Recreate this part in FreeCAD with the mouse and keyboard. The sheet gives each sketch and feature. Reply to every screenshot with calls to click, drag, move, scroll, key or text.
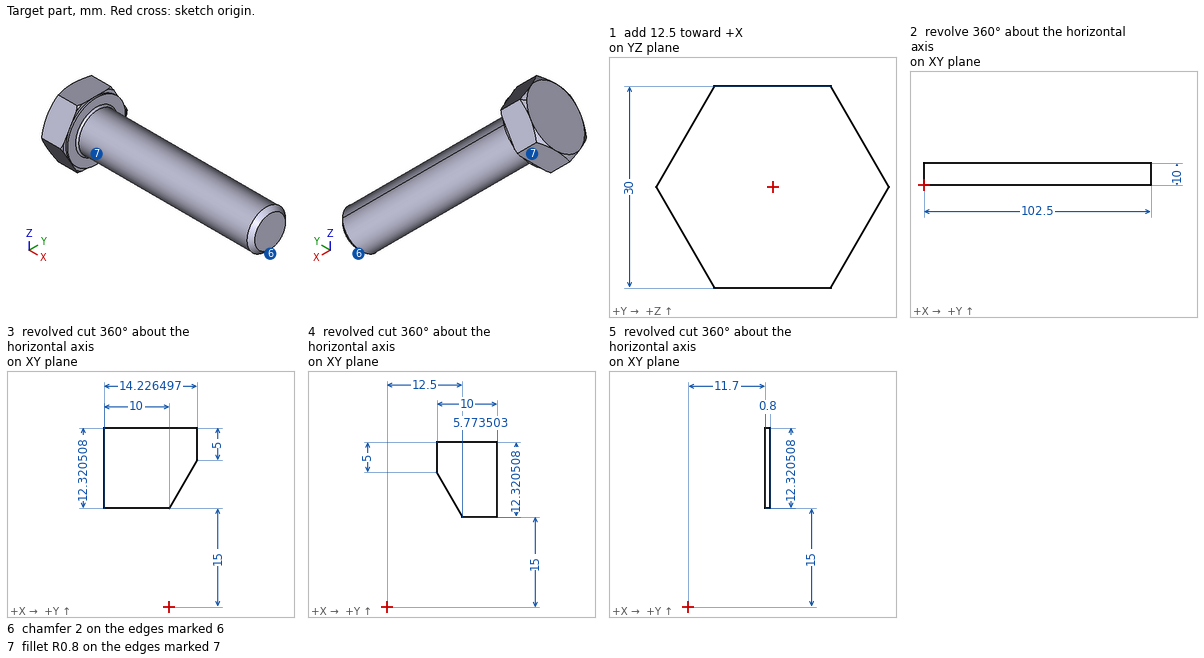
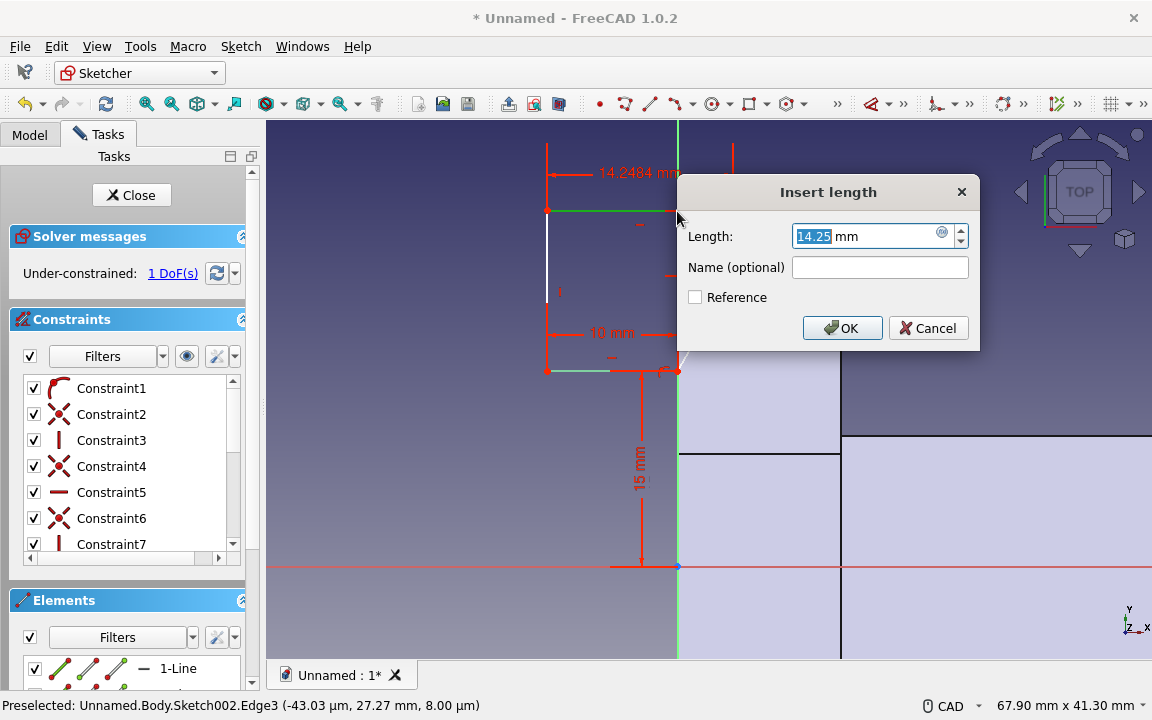
text(14.226497)
key(Return)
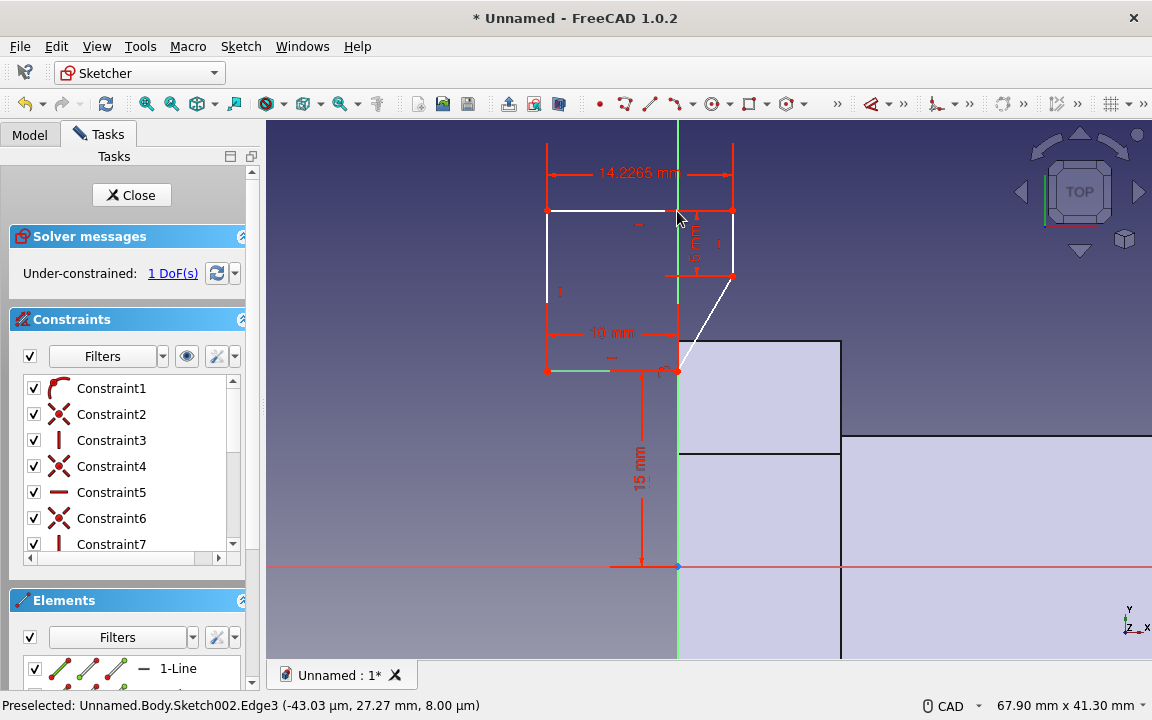
click(547, 259)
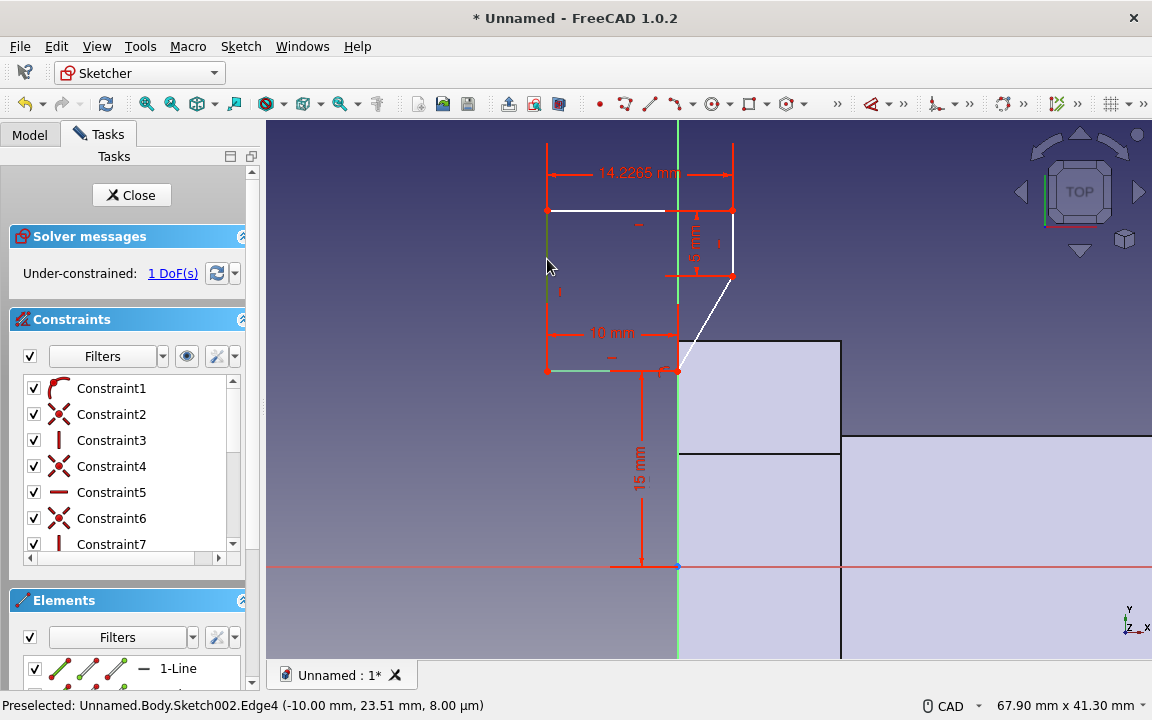
key(i)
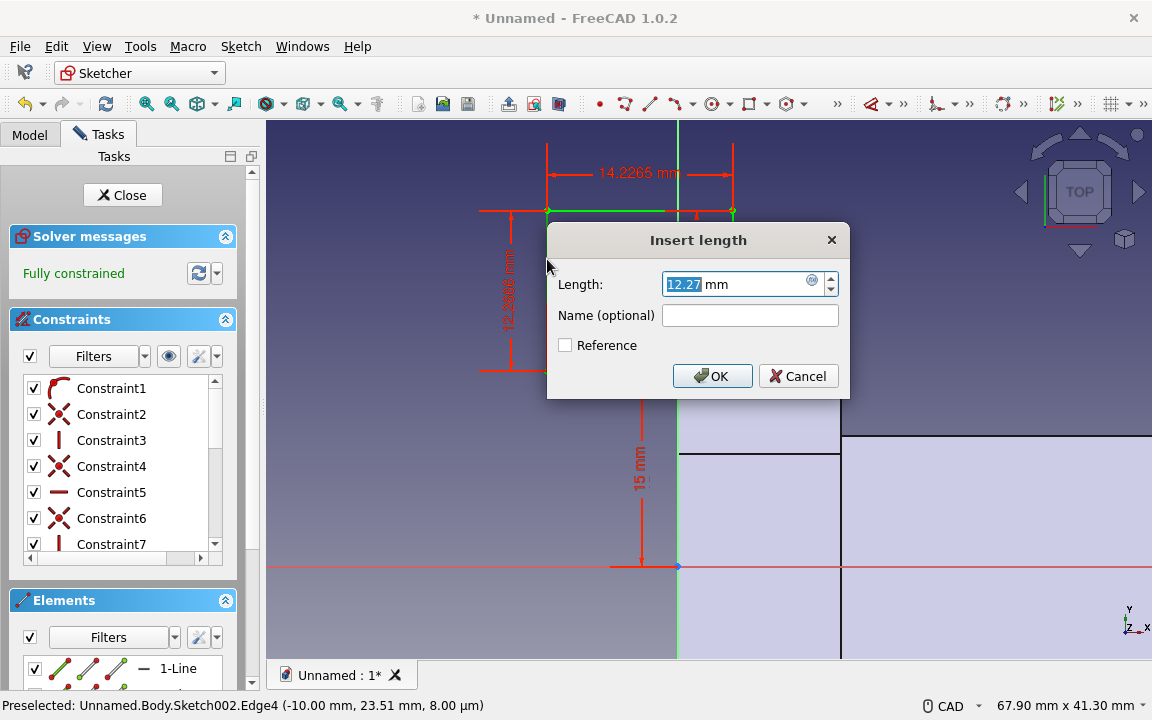
text(12.320508)
key(Return)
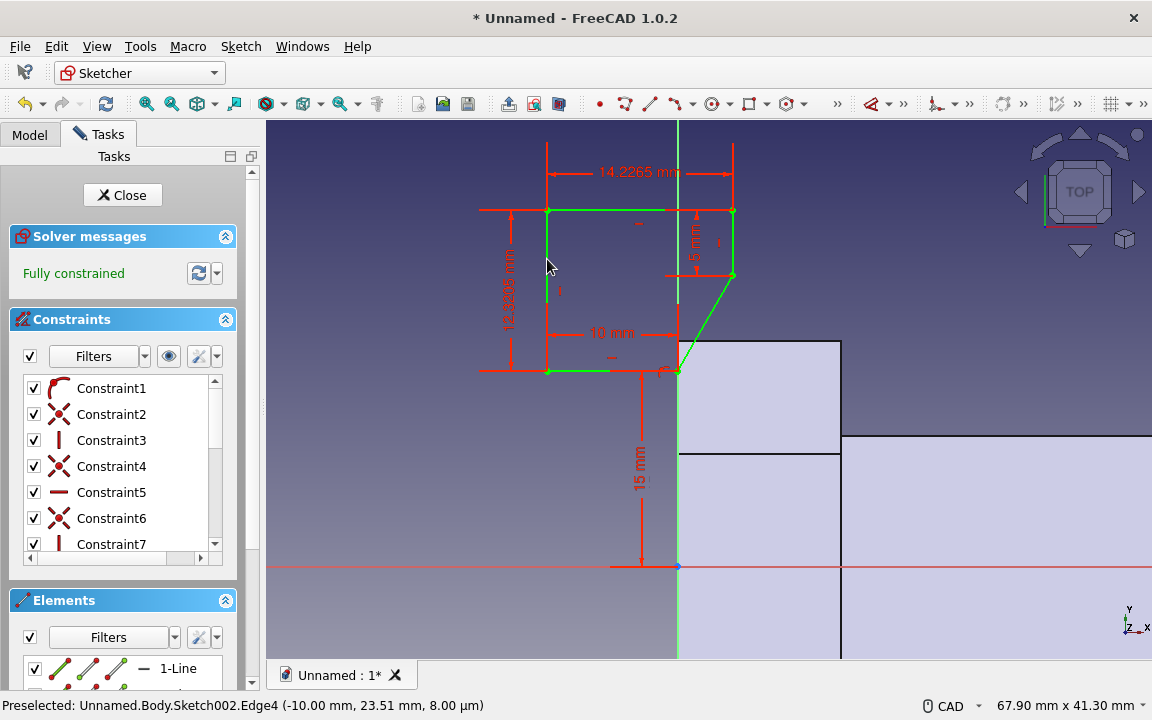
click(123, 195)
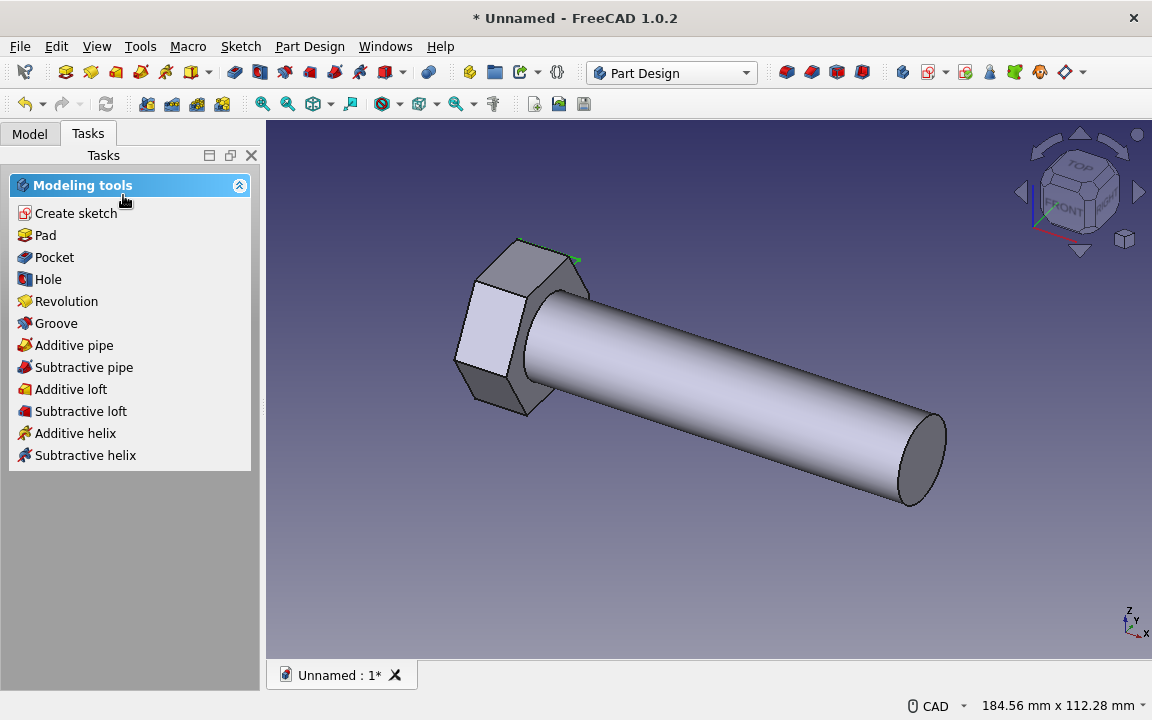
click(285, 72)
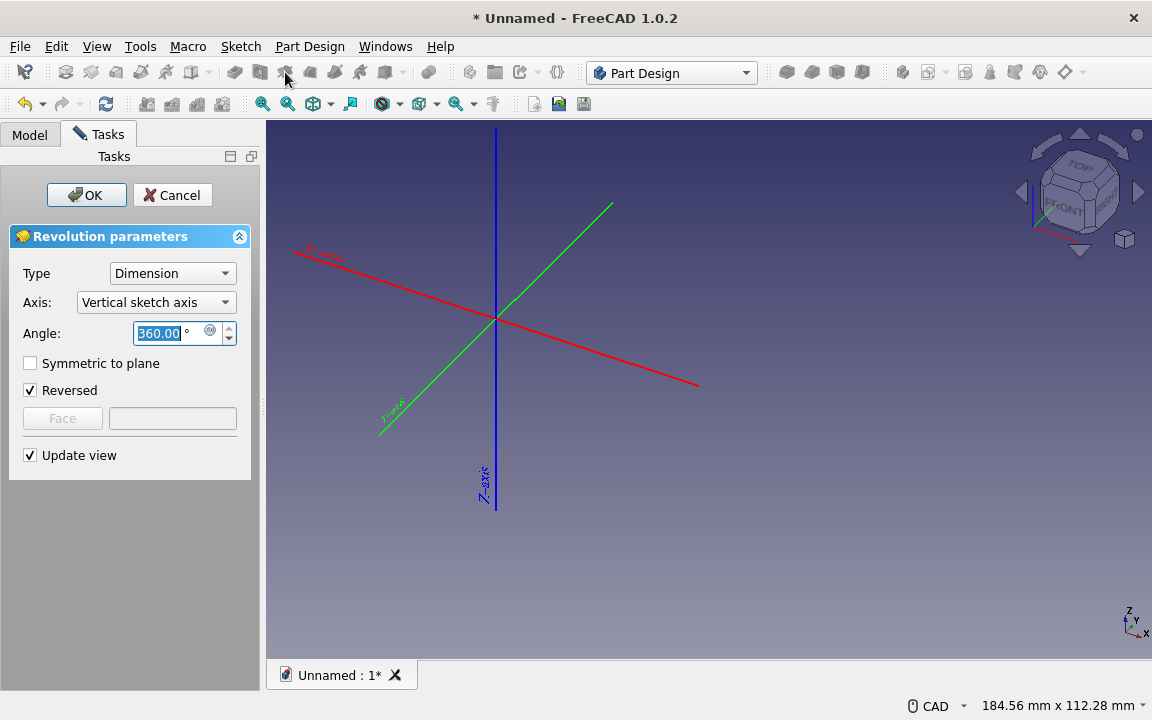
click(157, 302)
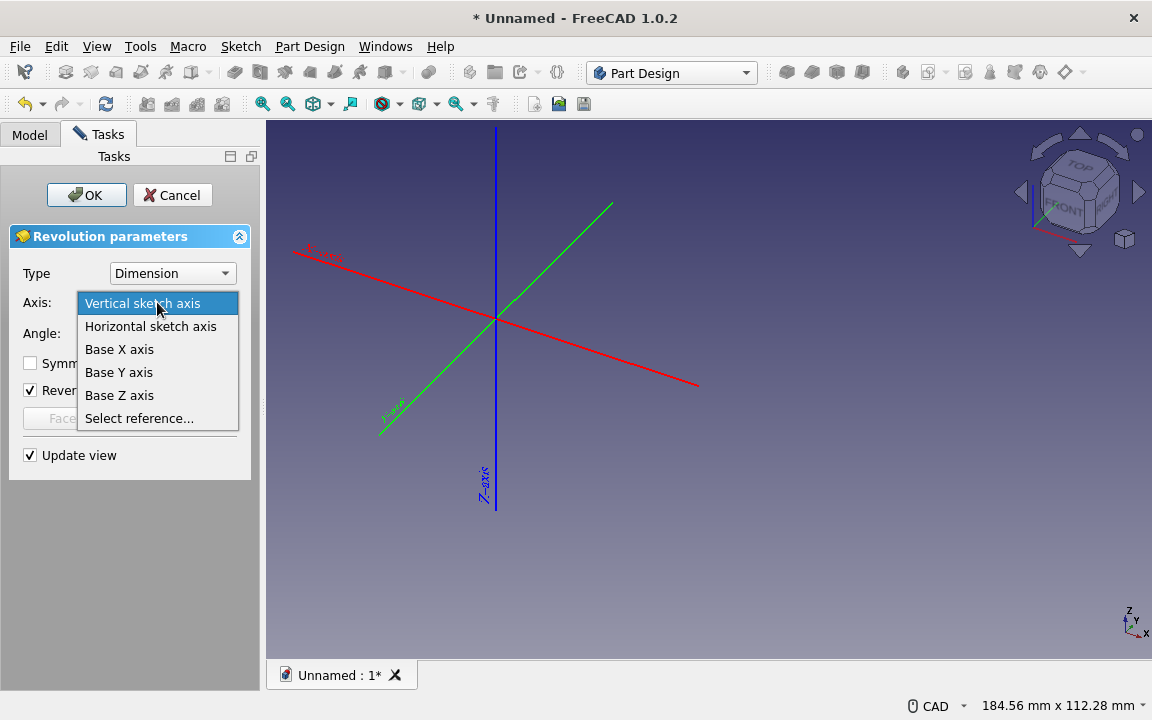
click(156, 326)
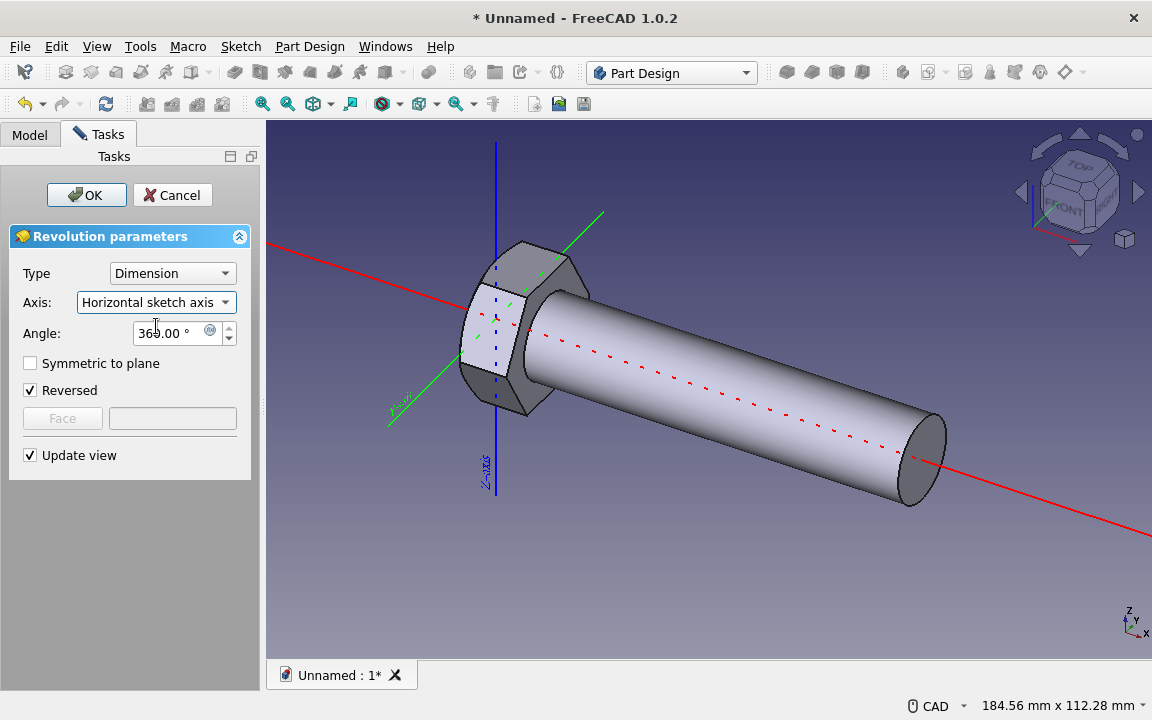
click(87, 195)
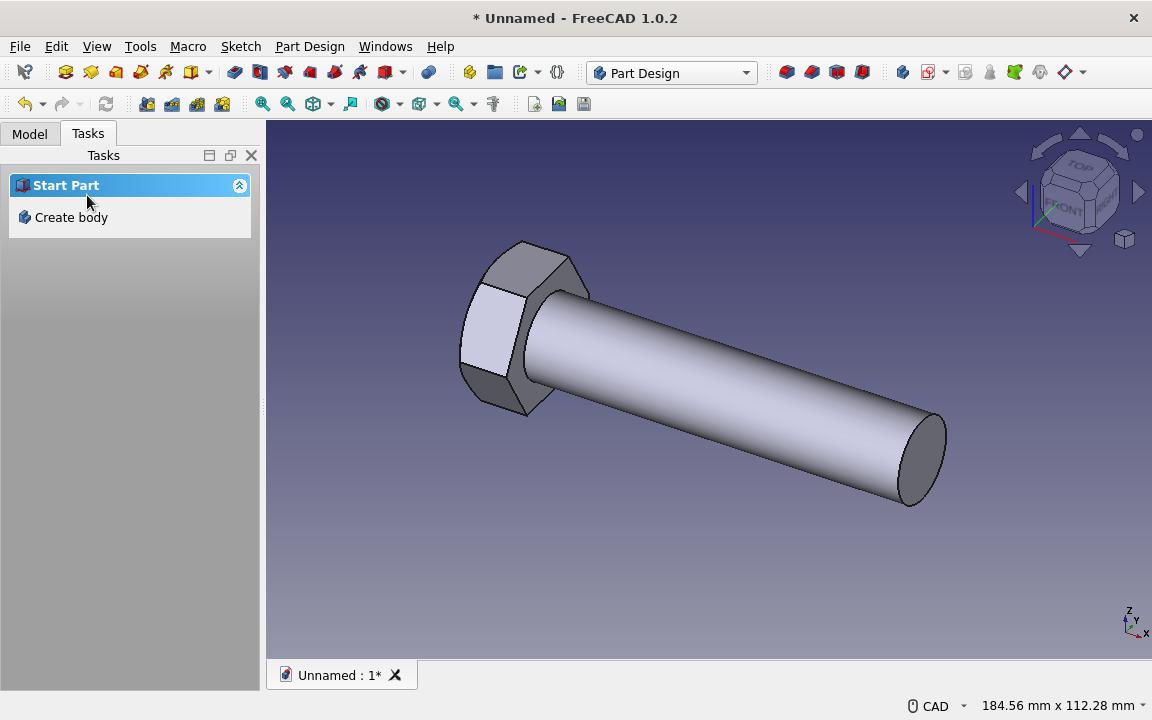
click(928, 72)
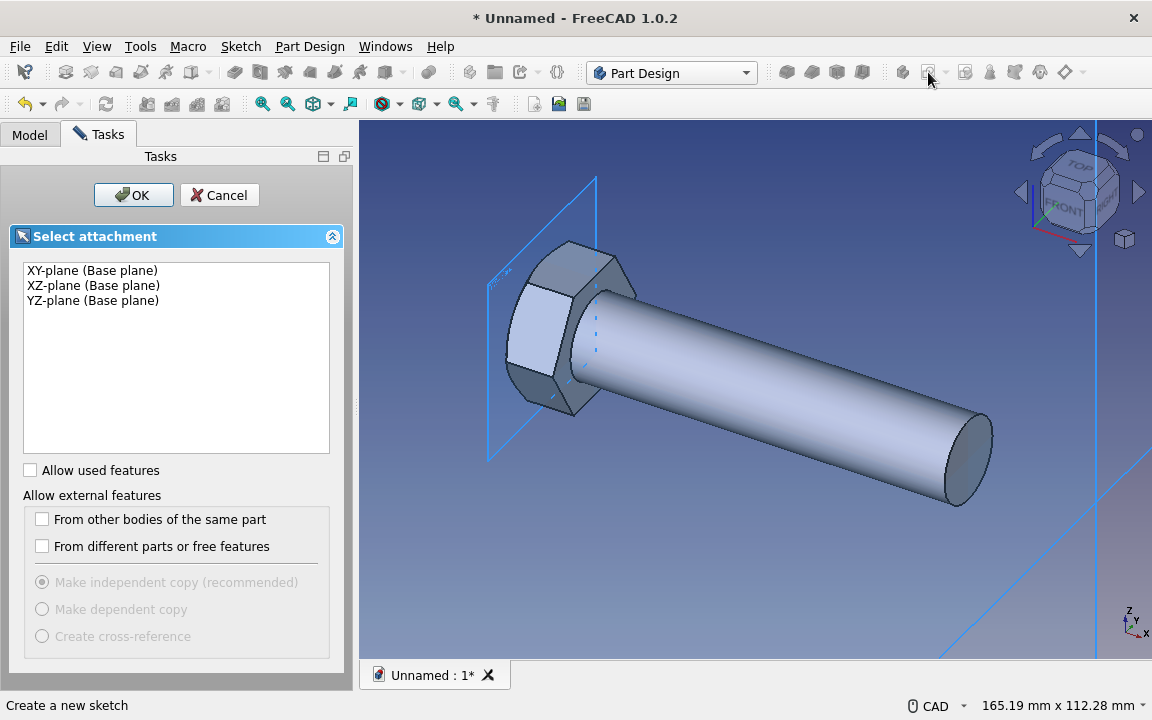
click(84, 270)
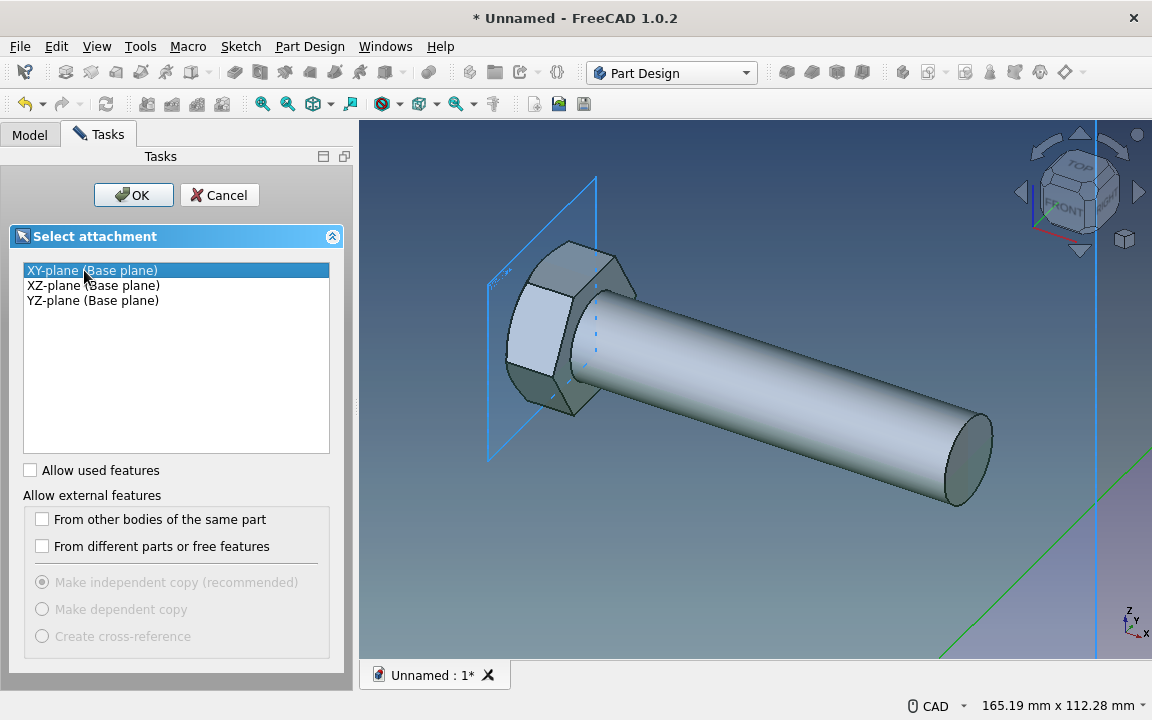
click(134, 195)